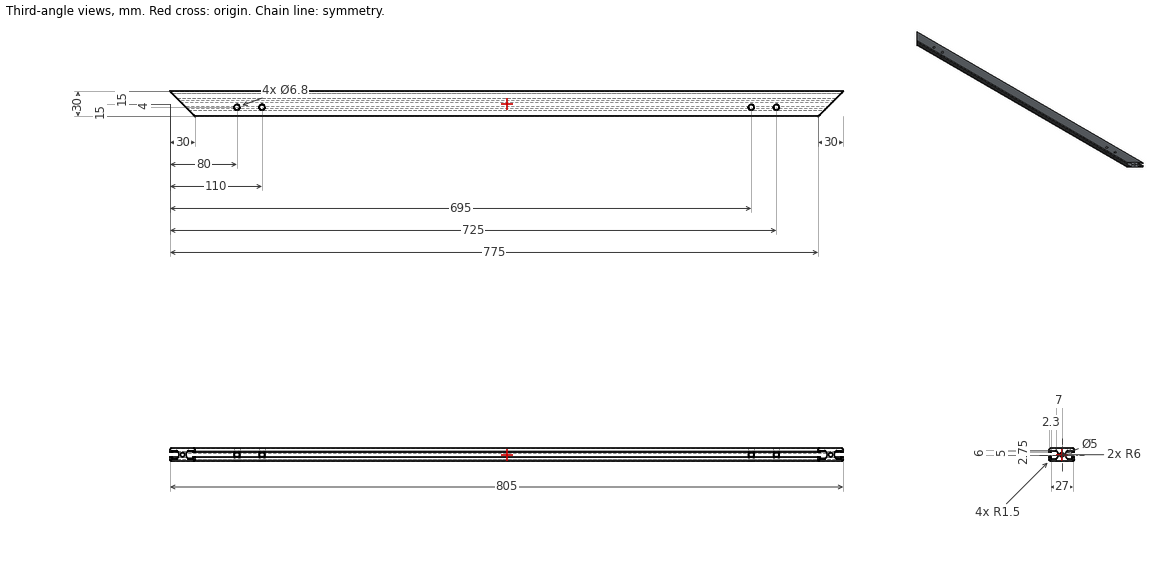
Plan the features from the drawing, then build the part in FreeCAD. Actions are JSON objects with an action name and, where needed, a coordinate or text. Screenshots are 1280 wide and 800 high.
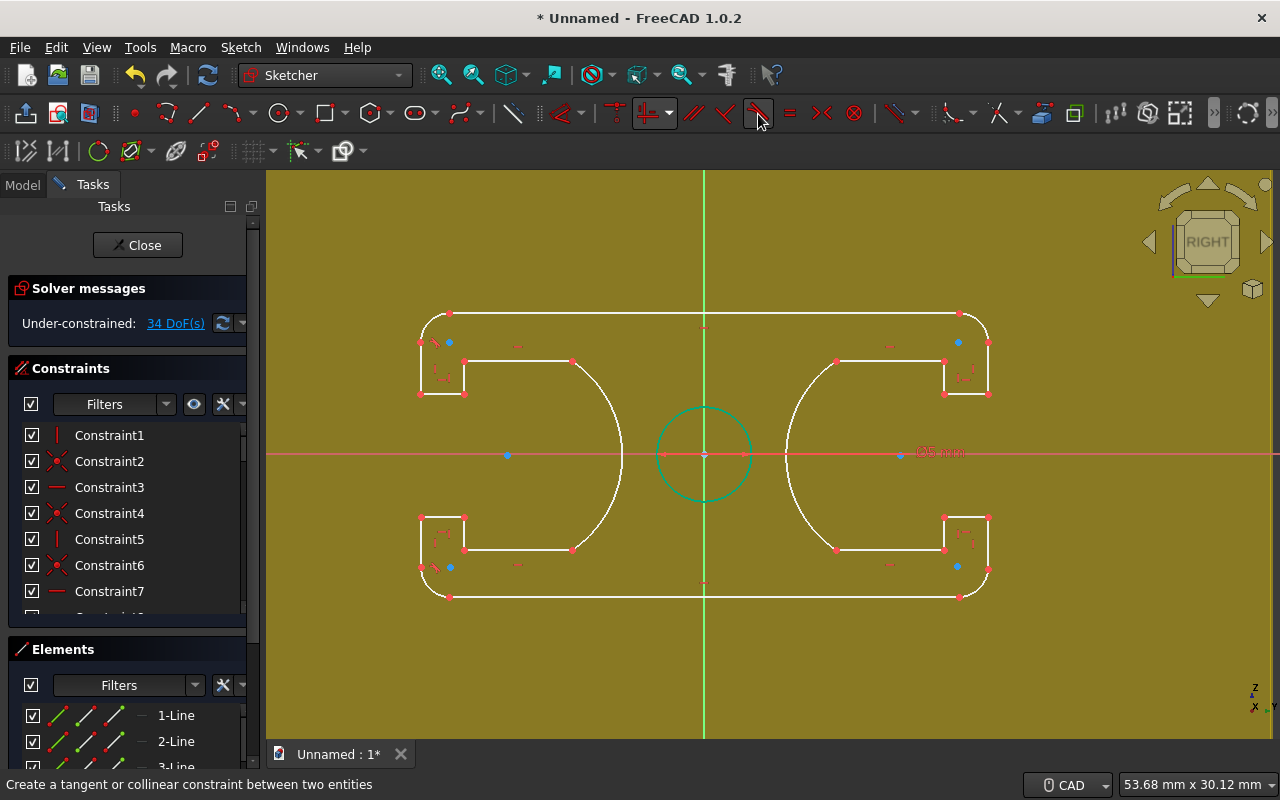
{"action": "left_click", "coordinate": [602, 597]}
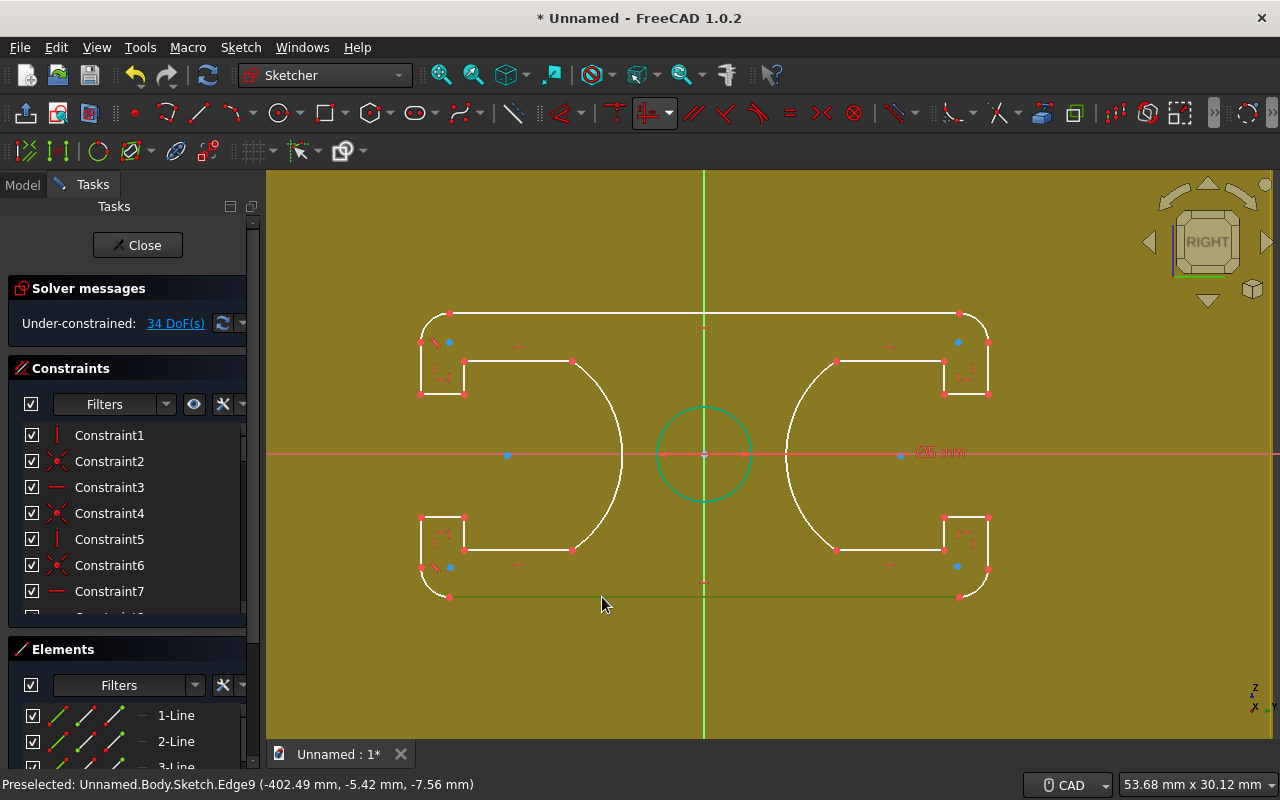
{"action": "left_click", "coordinate": [424, 581]}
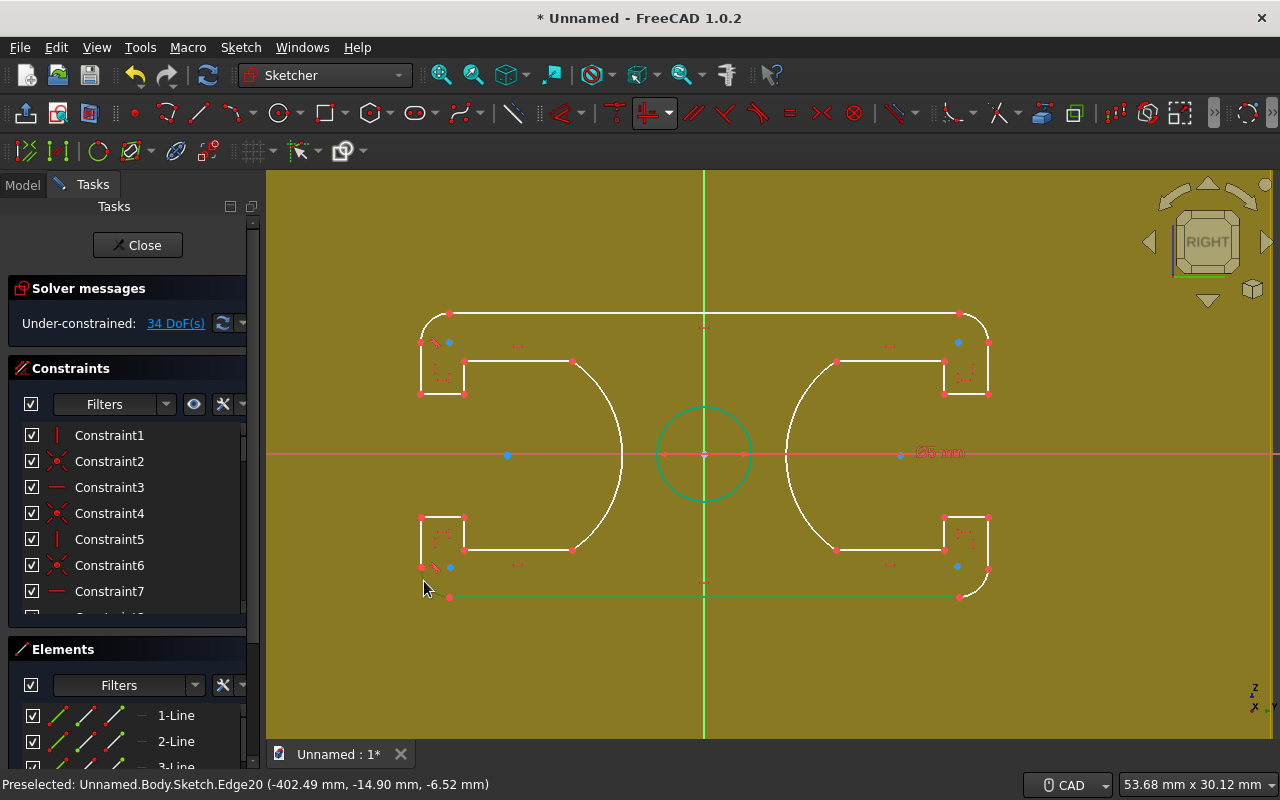
{"action": "left_click", "coordinate": [758, 114]}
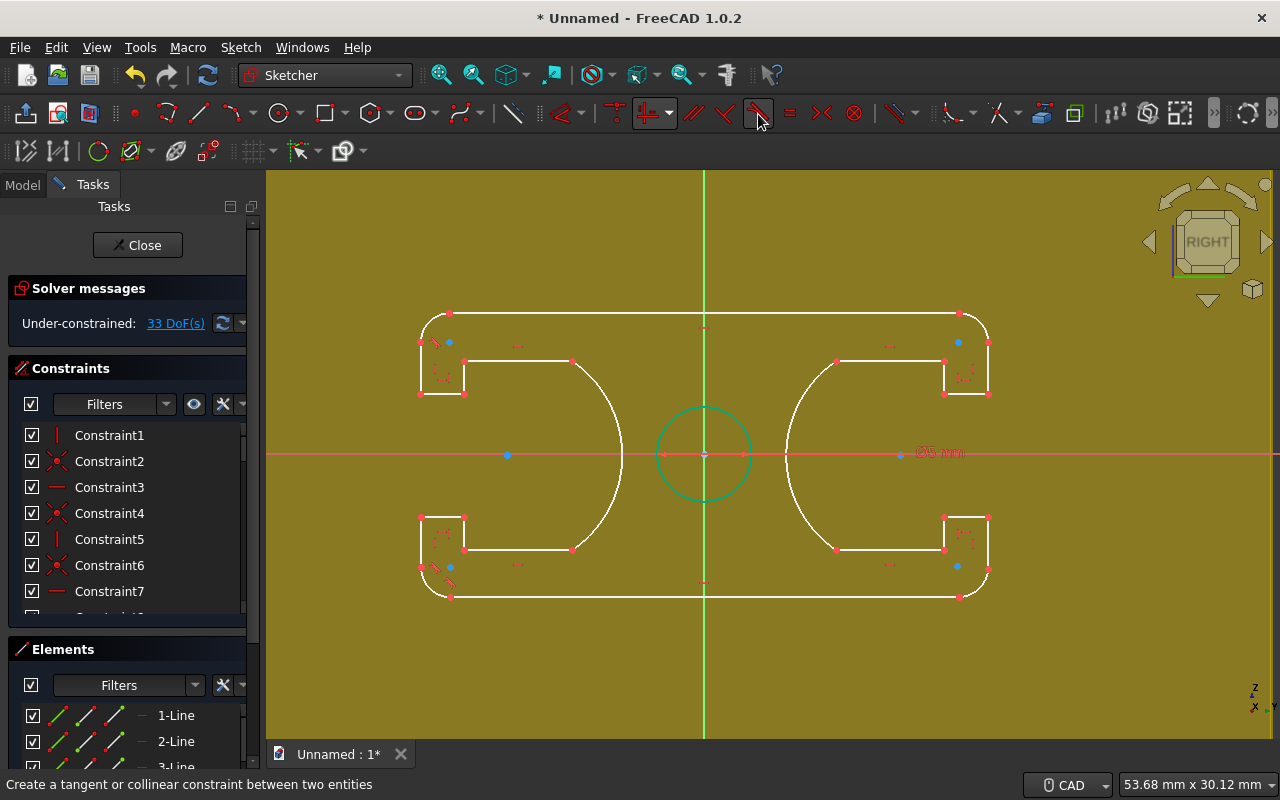
{"action": "left_click", "coordinate": [603, 597]}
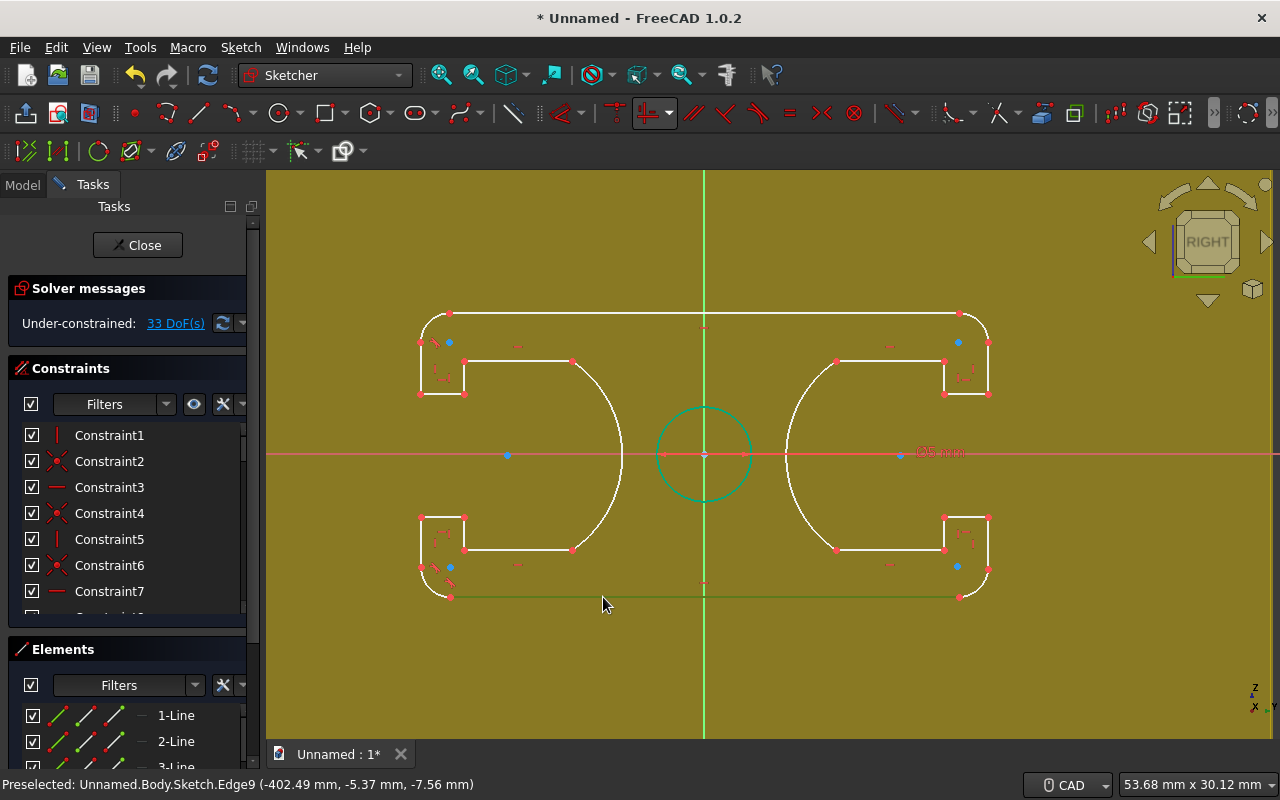
{"action": "left_click", "coordinate": [972, 594]}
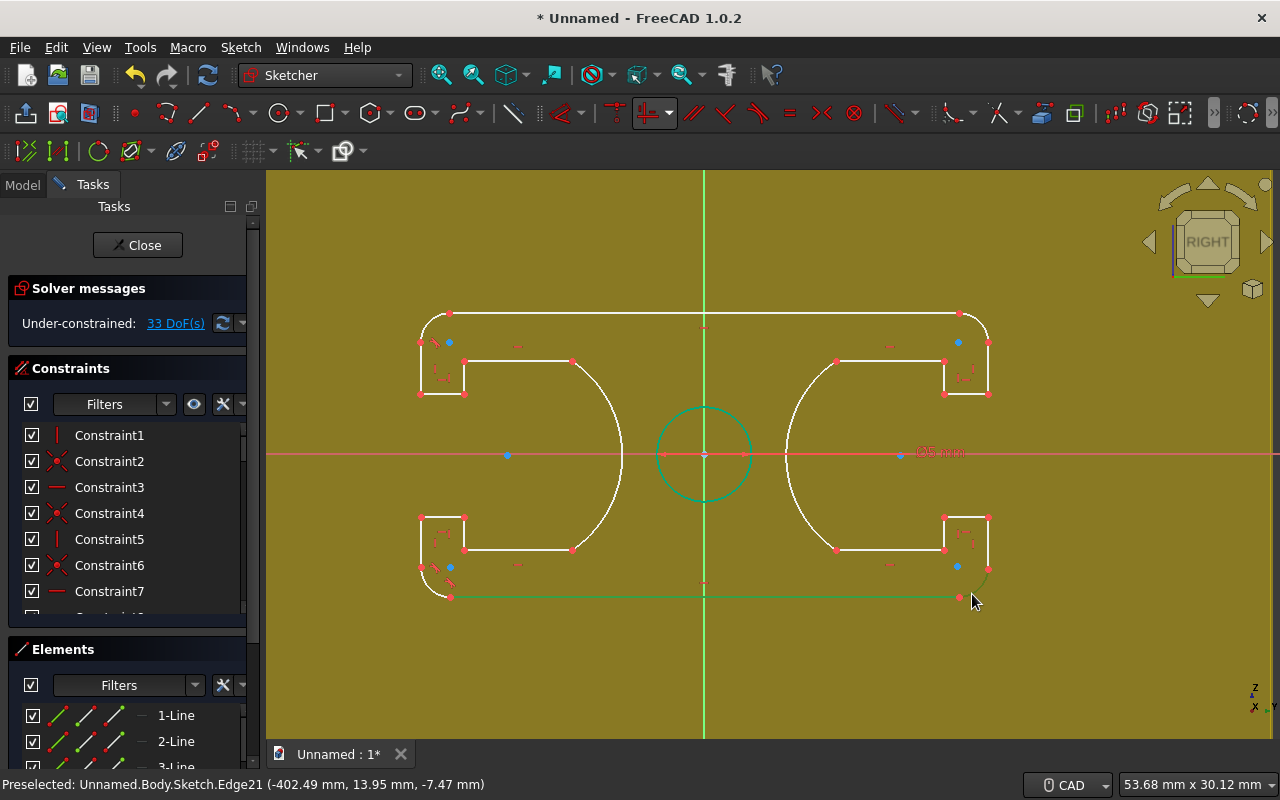
{"action": "left_click", "coordinate": [758, 114]}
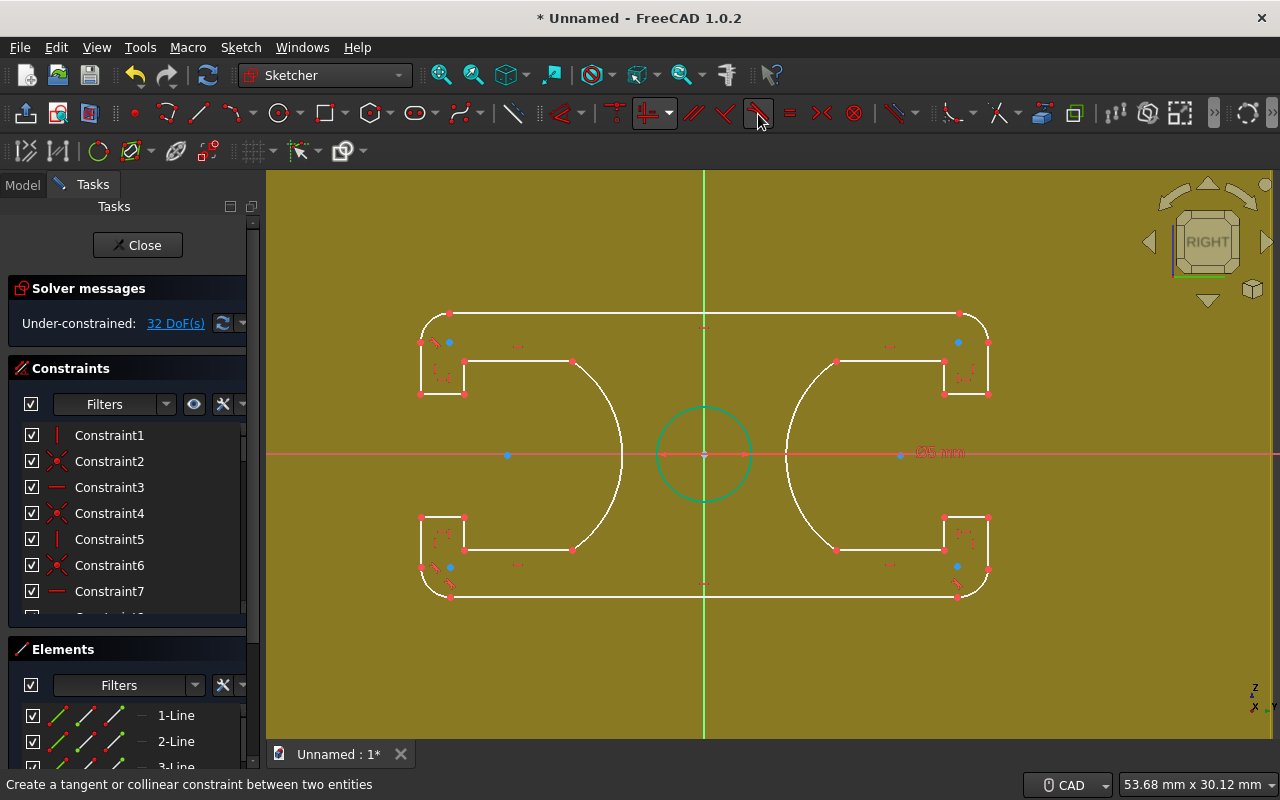
{"action": "left_click", "coordinate": [988, 554]}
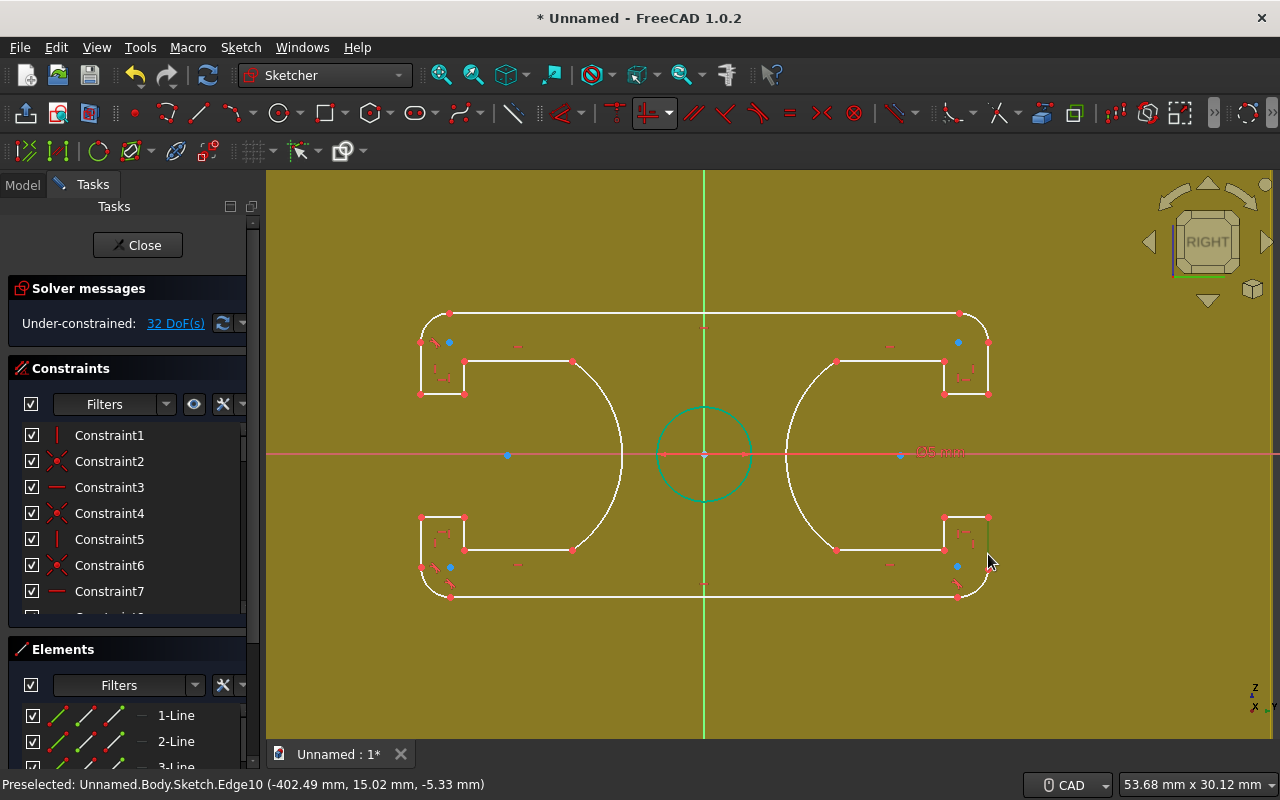
{"action": "left_click", "coordinate": [971, 594]}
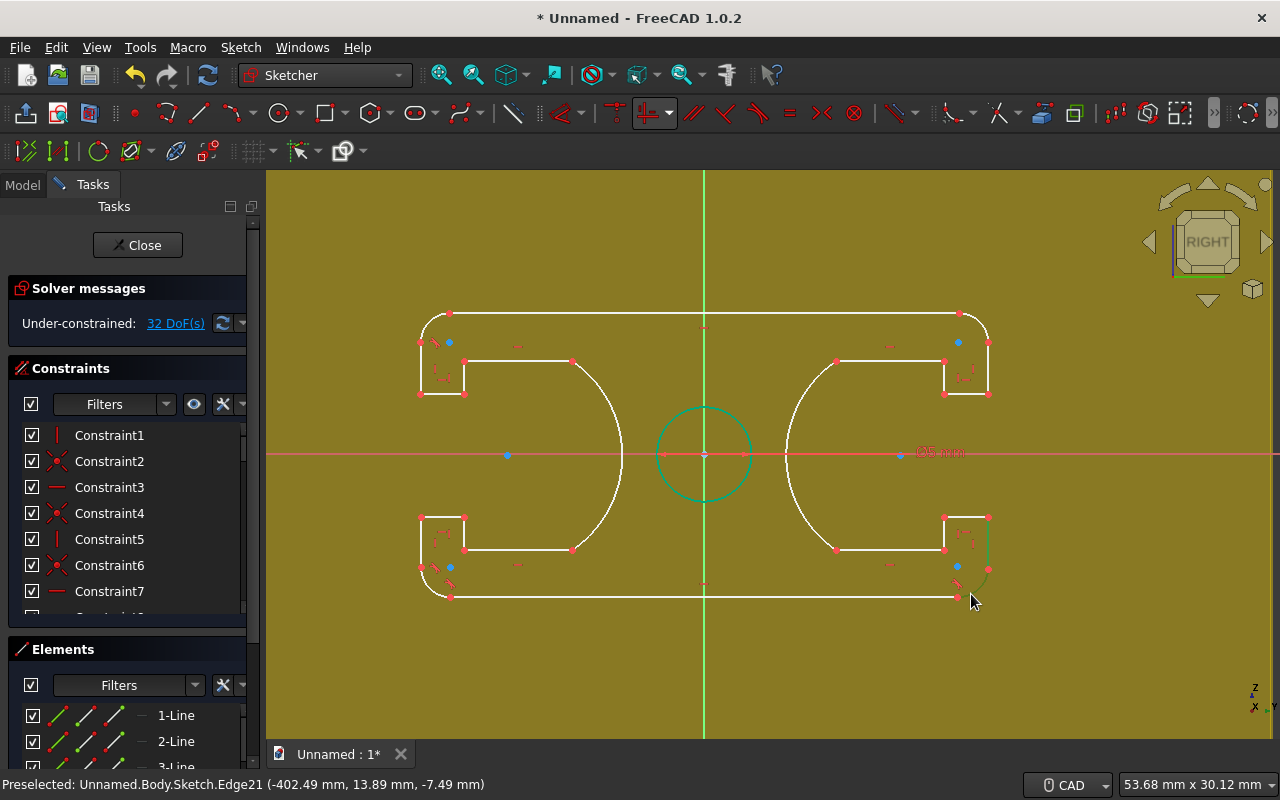
{"action": "left_click", "coordinate": [758, 114]}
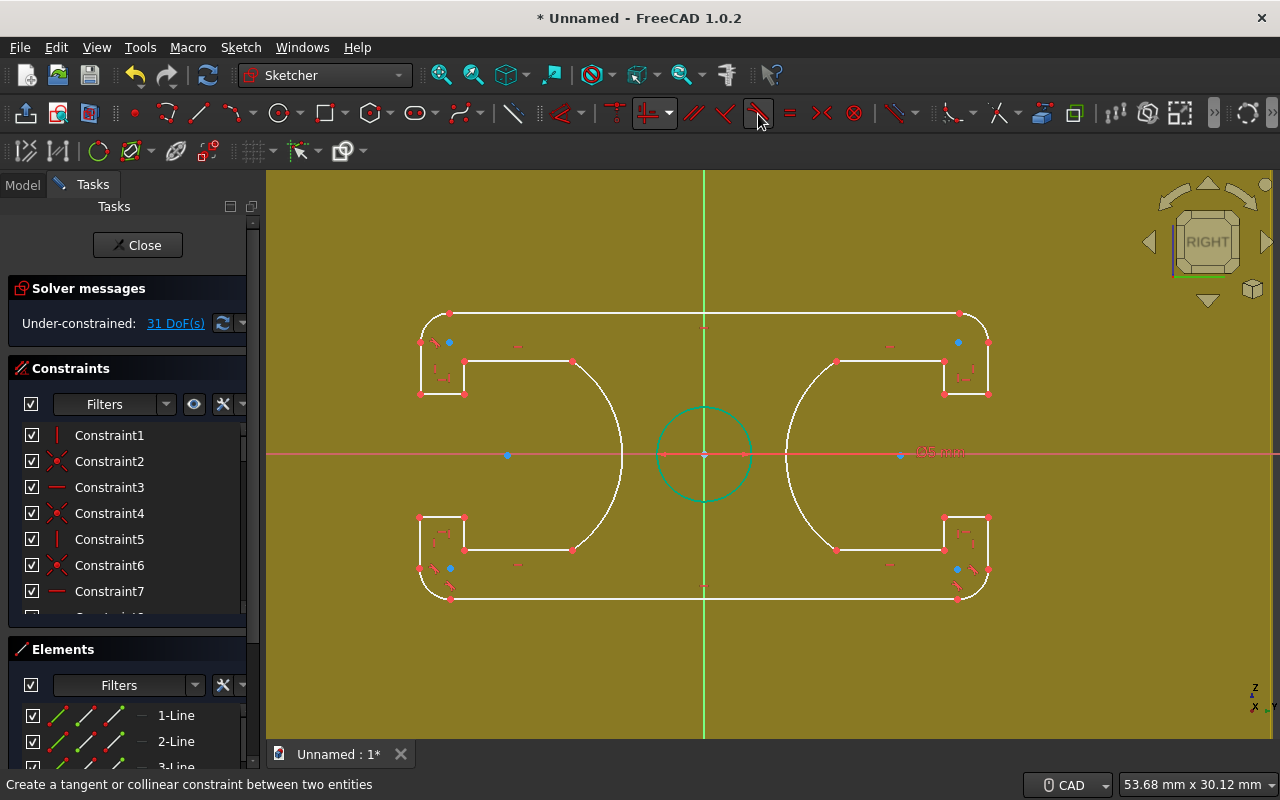
{"action": "left_click", "coordinate": [988, 379]}